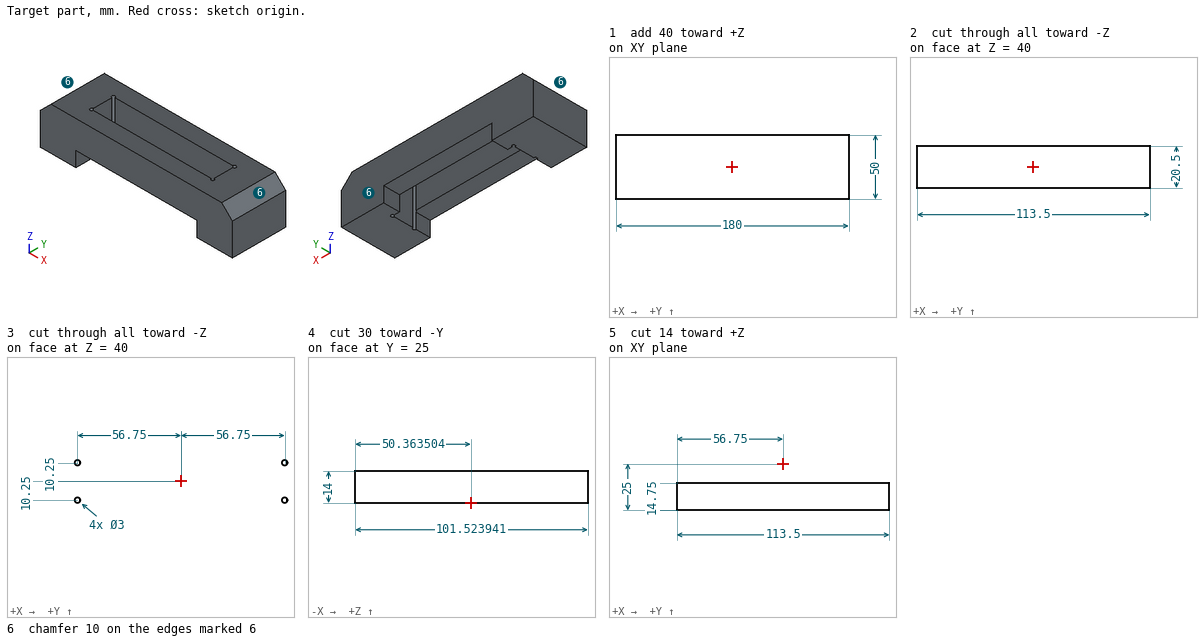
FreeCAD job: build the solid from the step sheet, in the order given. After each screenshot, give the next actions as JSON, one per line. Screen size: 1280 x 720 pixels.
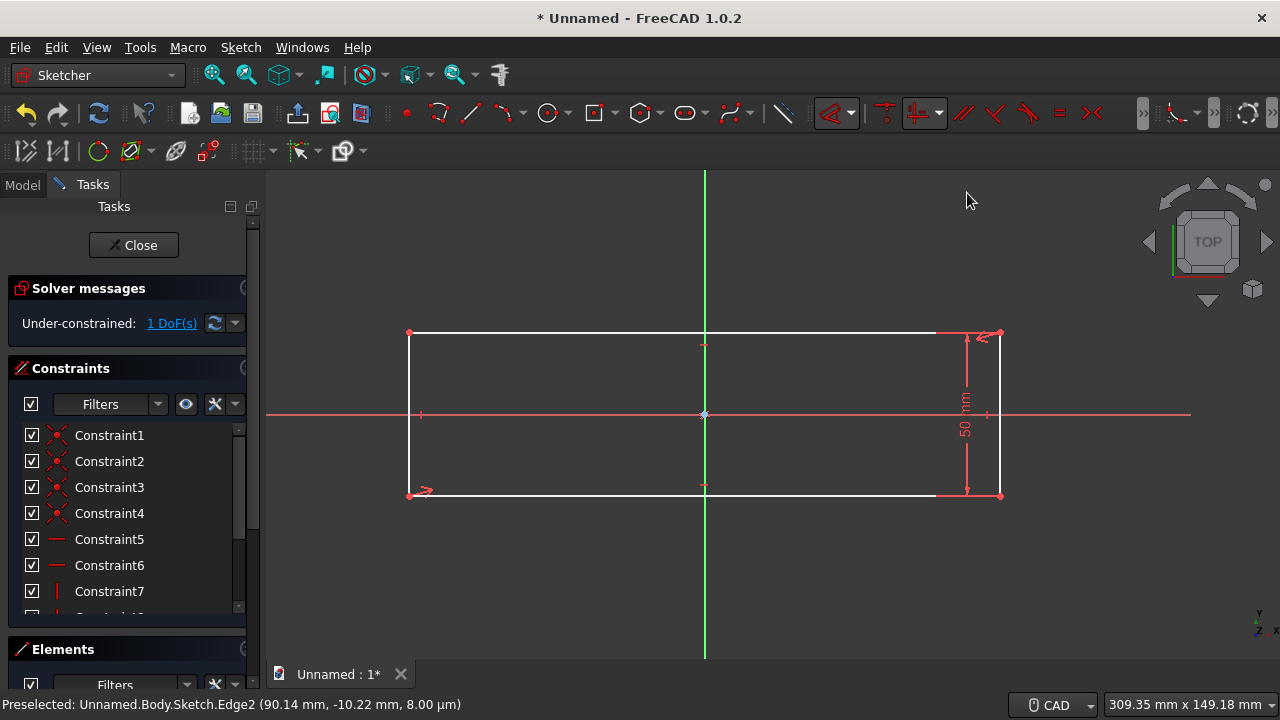
{"action": "left_click", "coordinate": [586, 496]}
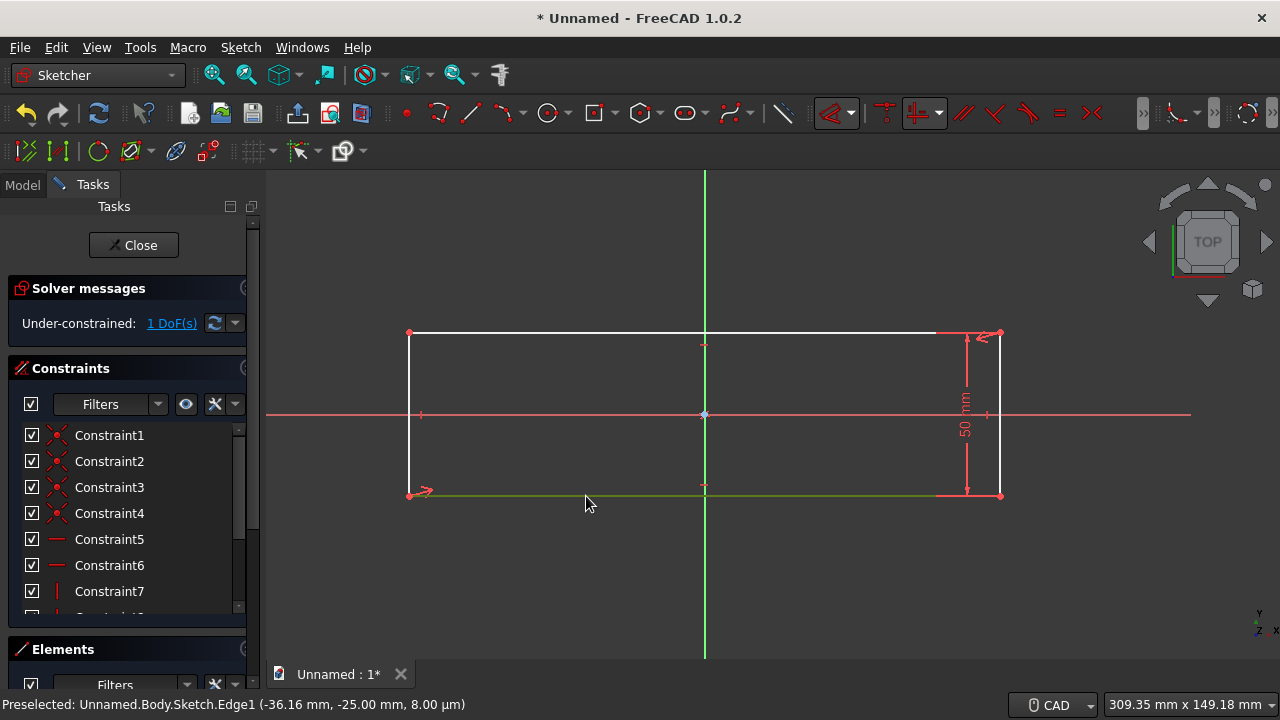
{"action": "left_click", "coordinate": [854, 114]}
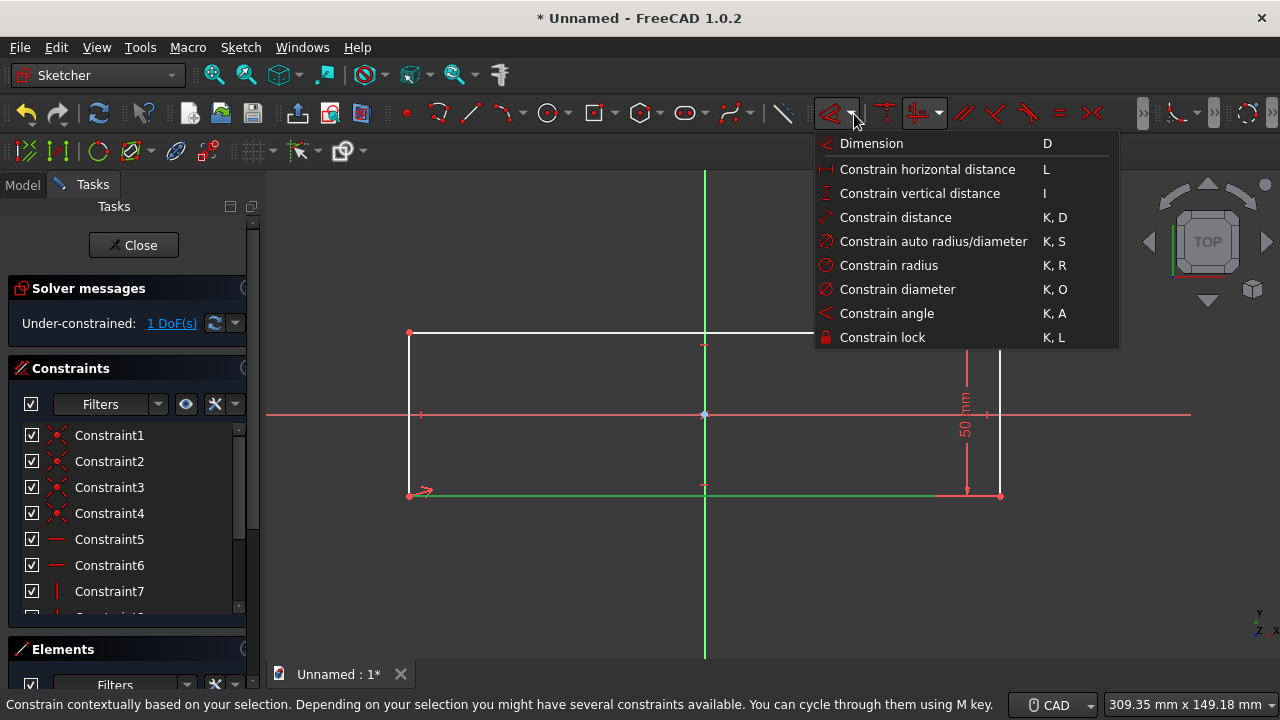
{"action": "left_click", "coordinate": [967, 169]}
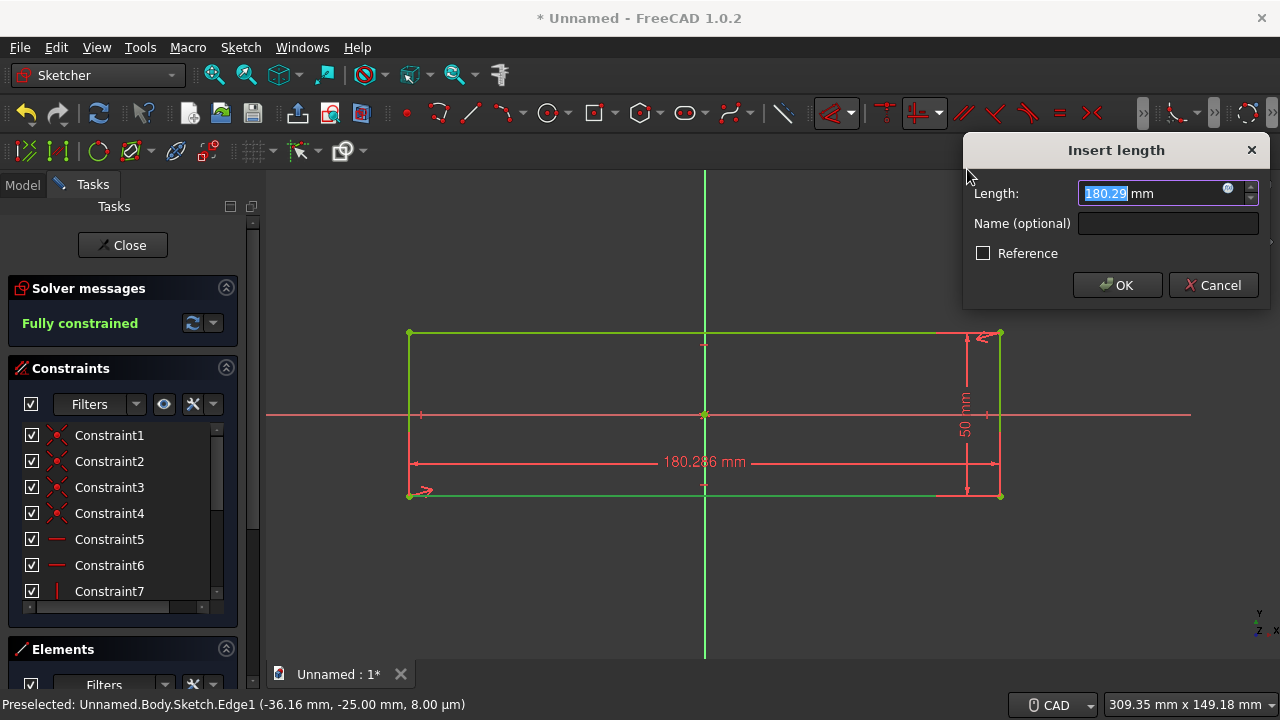
{"action": "type", "text": "180"}
{"action": "key", "text": "Return"}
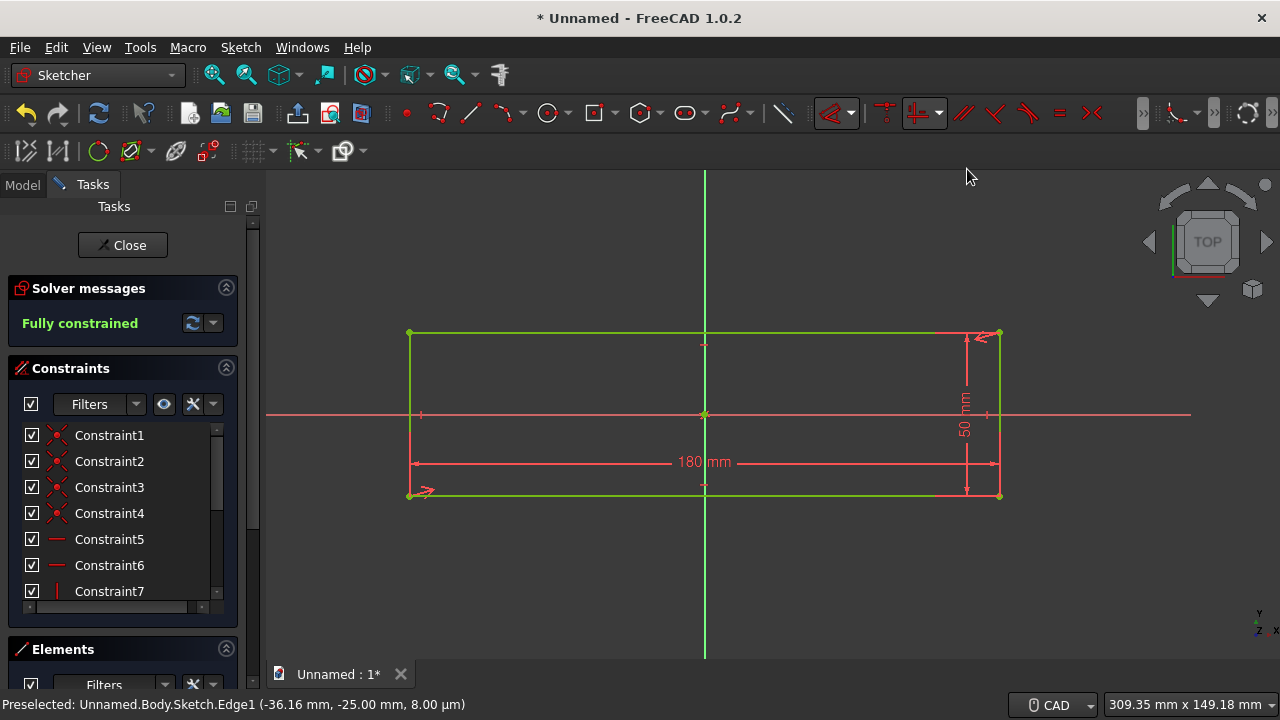
{"action": "left_click", "coordinate": [123, 245]}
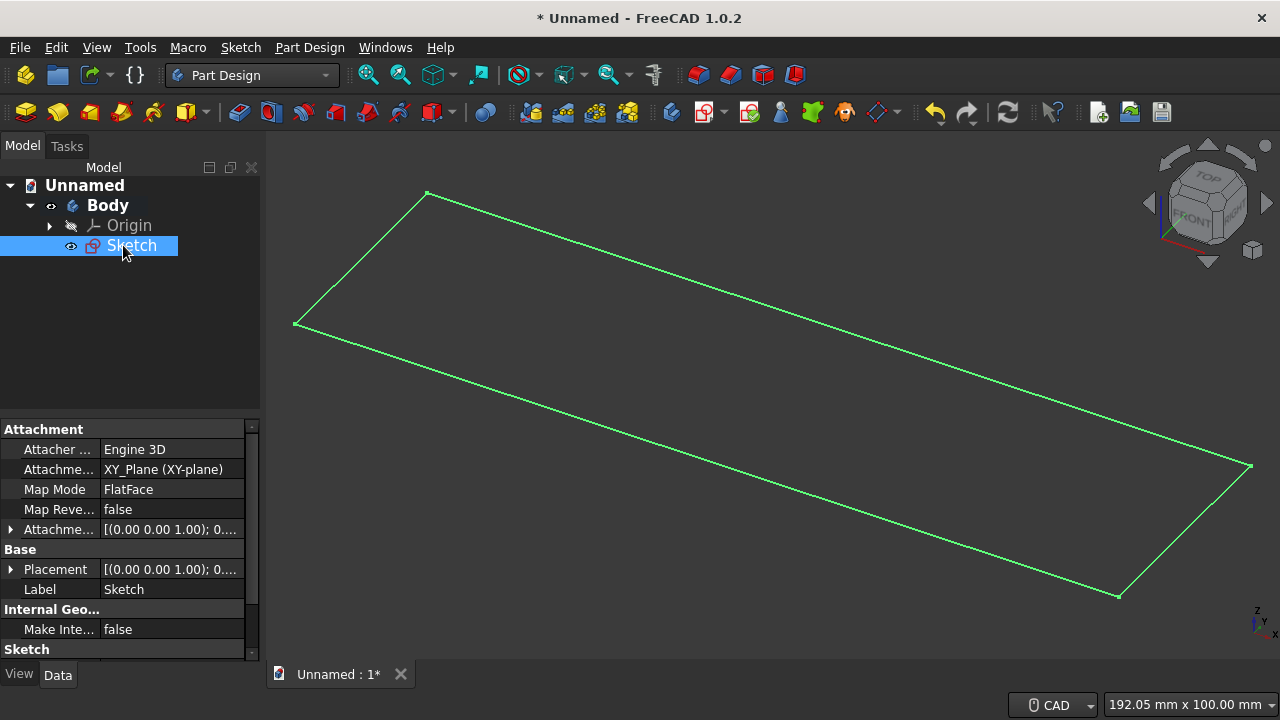
{"action": "left_click", "coordinate": [26, 112]}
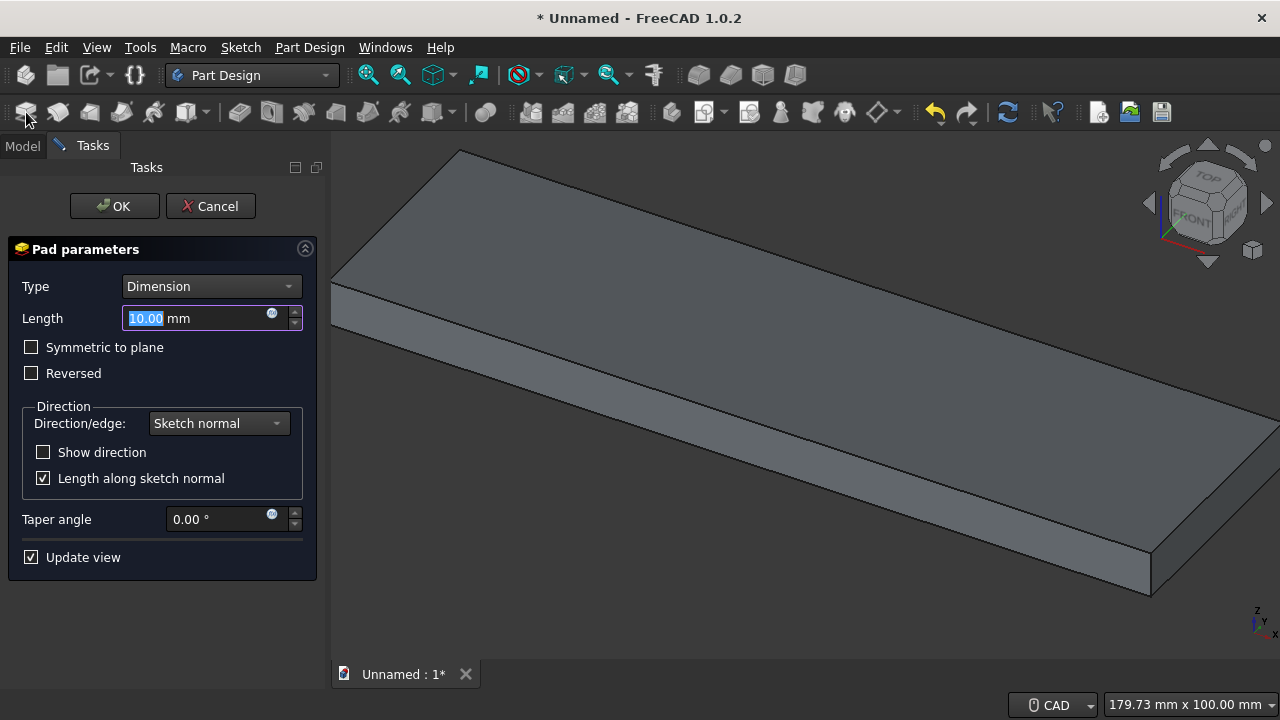
{"action": "type", "text": "40"}
{"action": "key", "text": "Tab"}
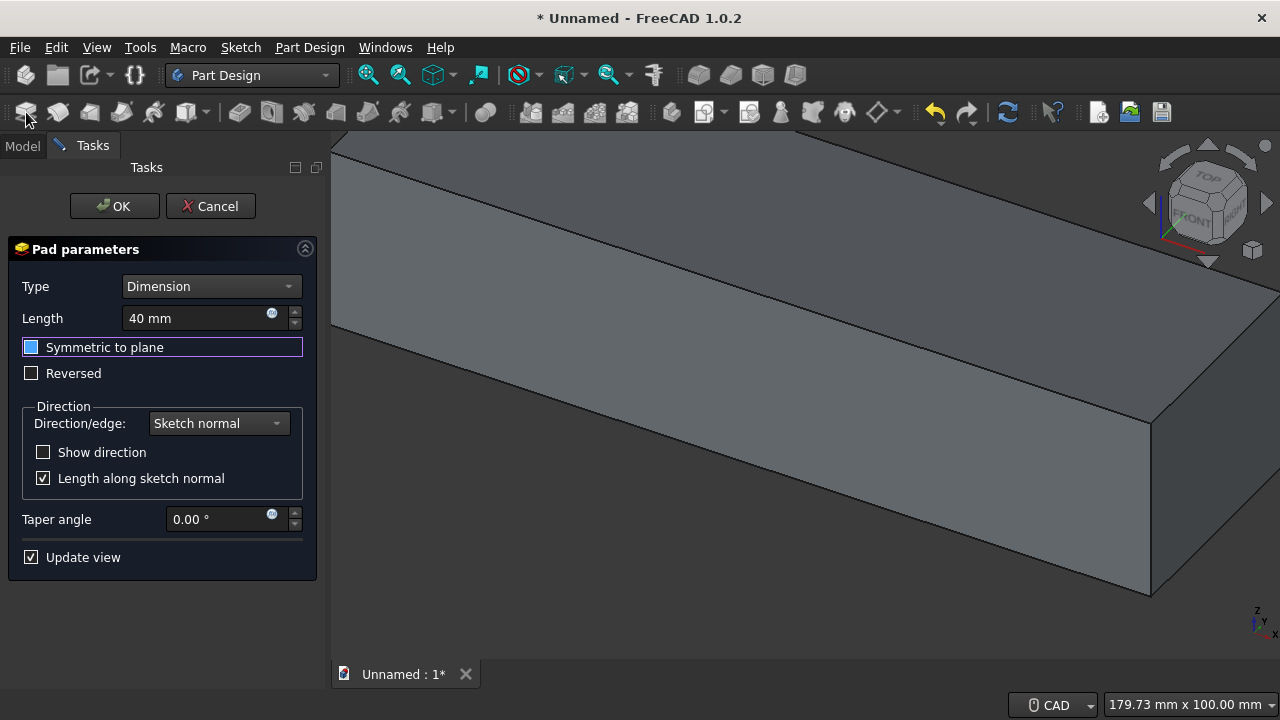
{"action": "left_click", "coordinate": [115, 206]}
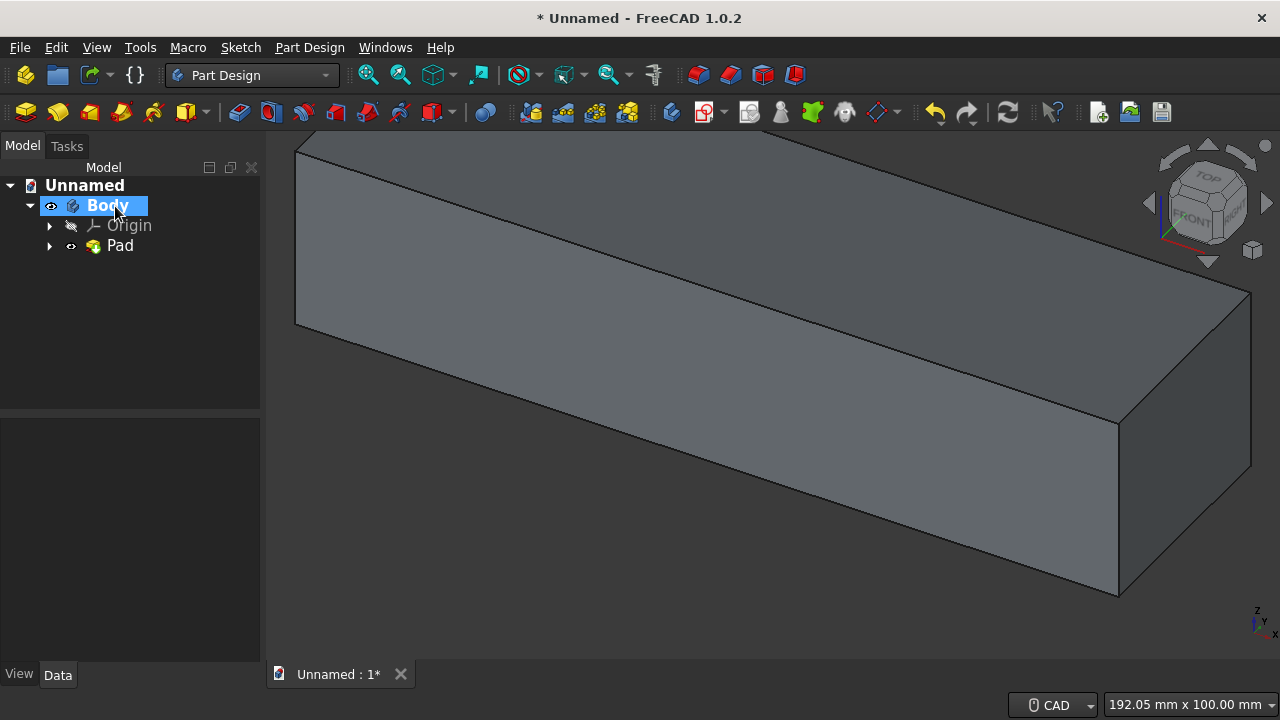
{"action": "left_click", "coordinate": [370, 76]}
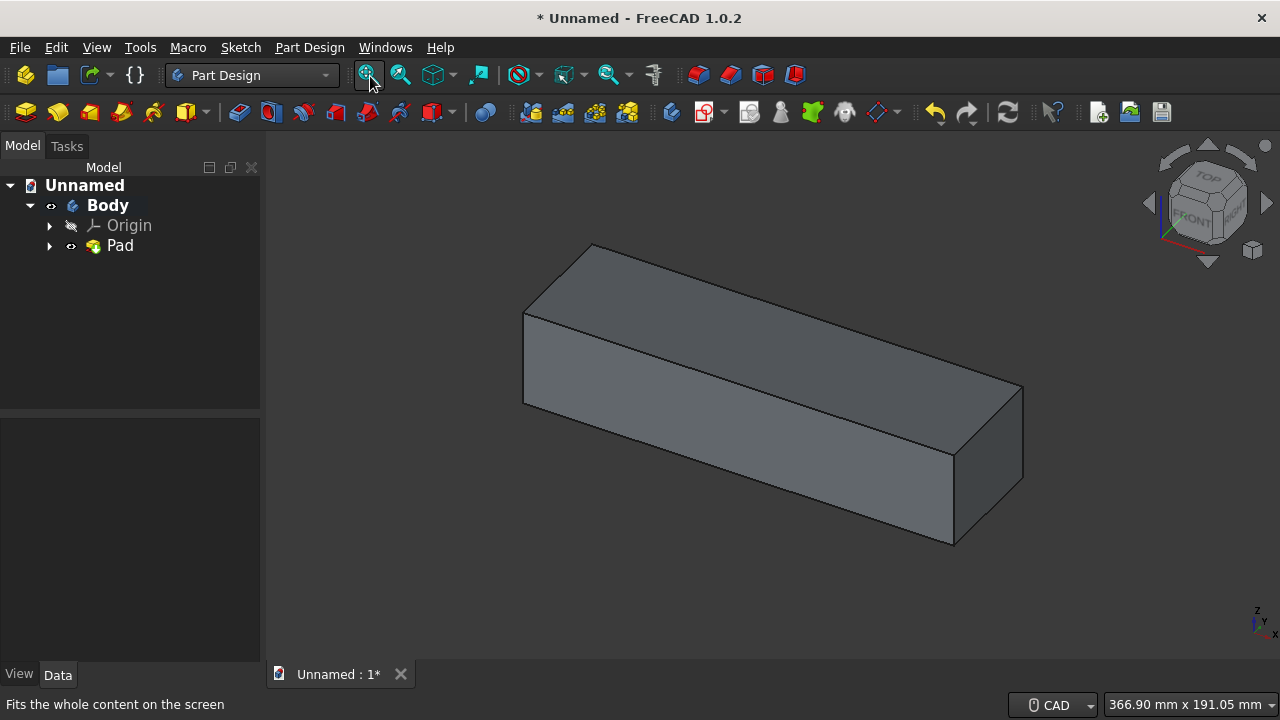
{"action": "left_click", "coordinate": [896, 389]}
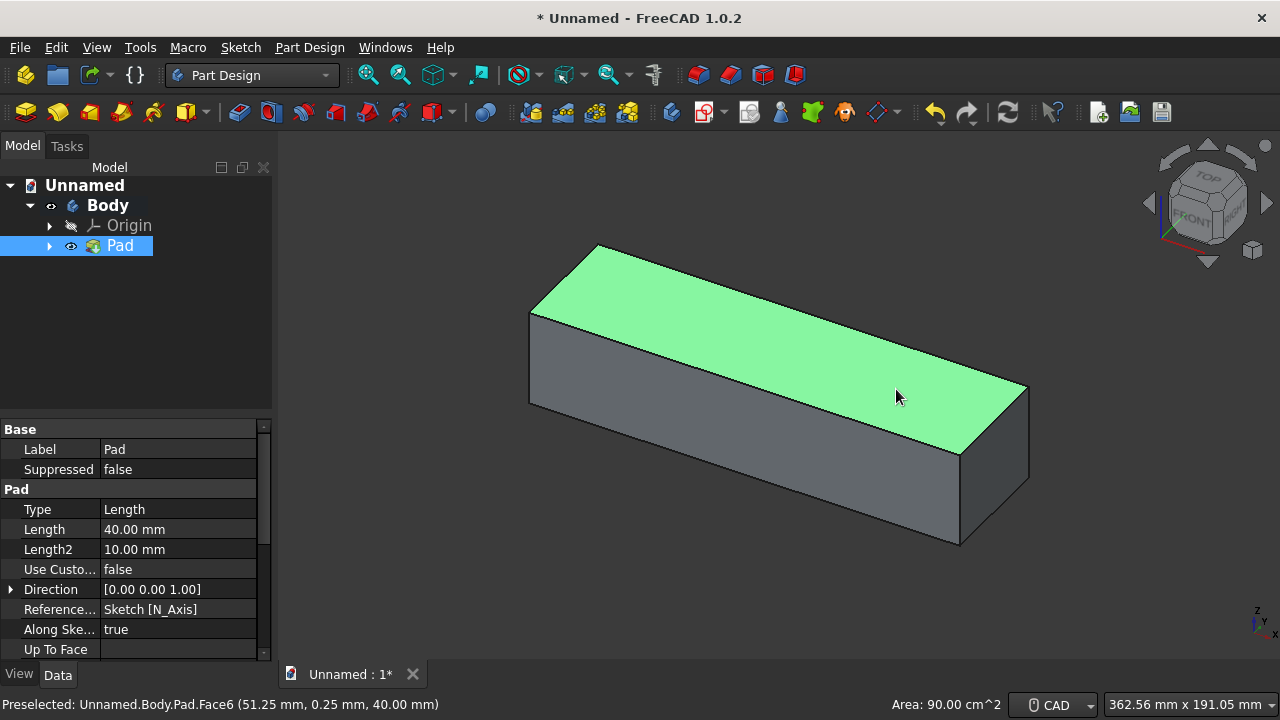
{"action": "left_click", "coordinate": [704, 112]}